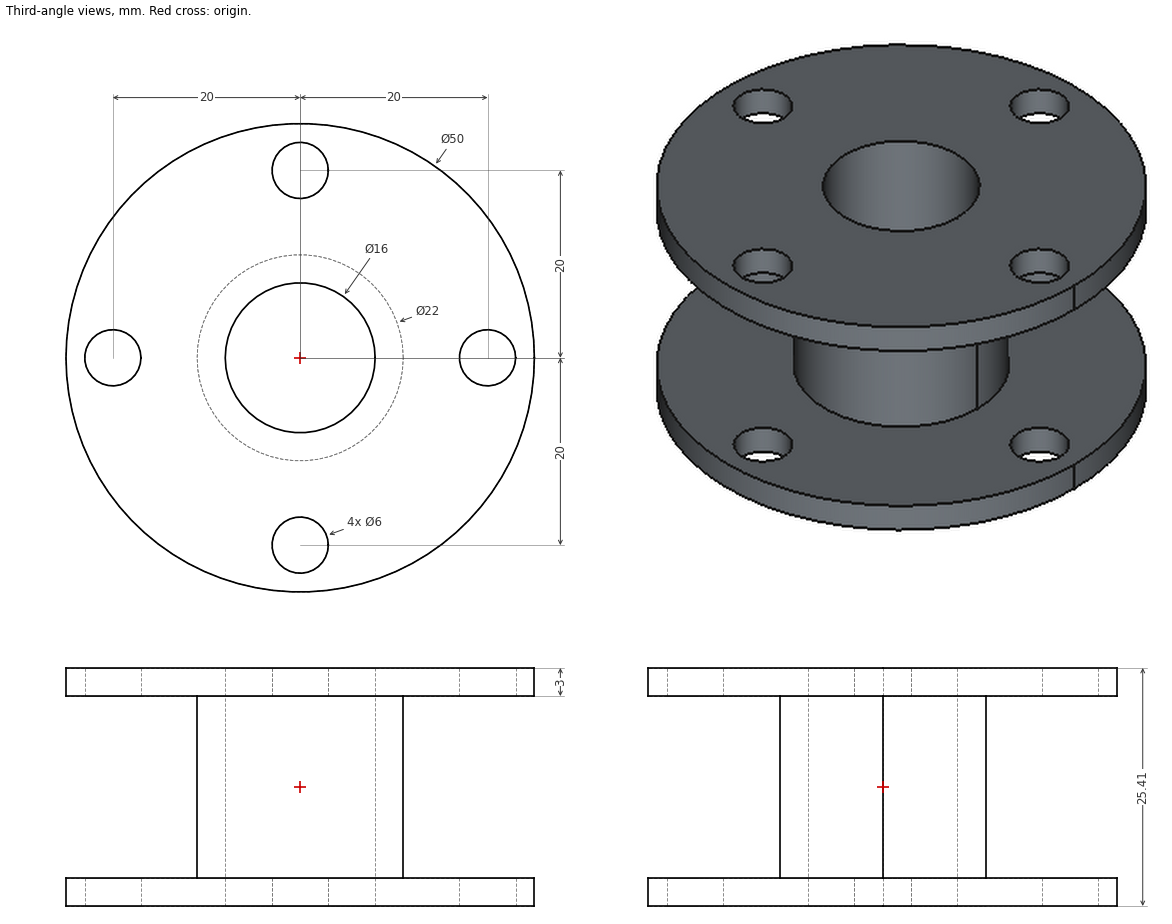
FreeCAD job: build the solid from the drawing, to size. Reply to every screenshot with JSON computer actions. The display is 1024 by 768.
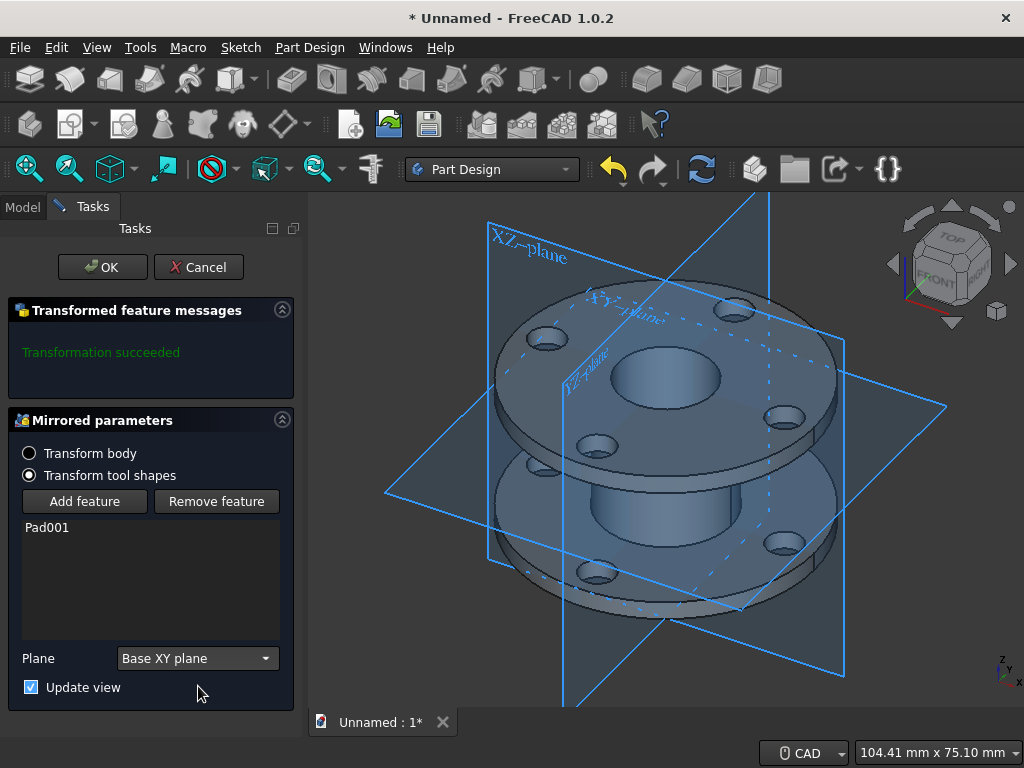
{"action": "left_click", "coordinate": [103, 267]}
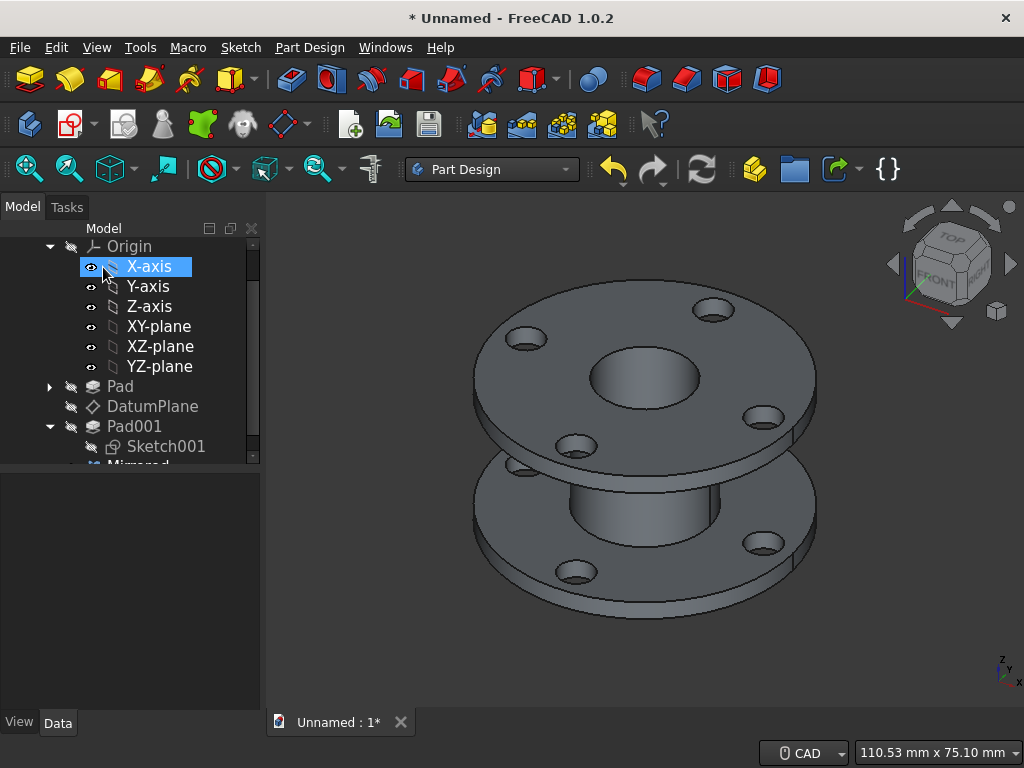
{"action": "key", "text": "0"}